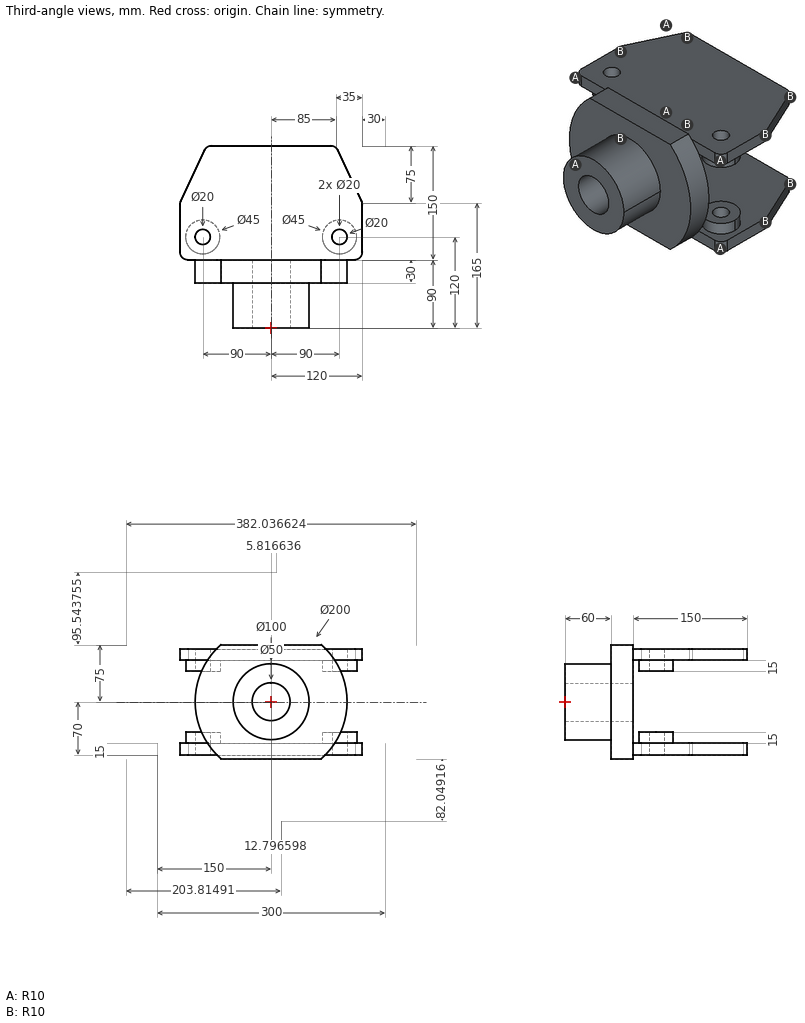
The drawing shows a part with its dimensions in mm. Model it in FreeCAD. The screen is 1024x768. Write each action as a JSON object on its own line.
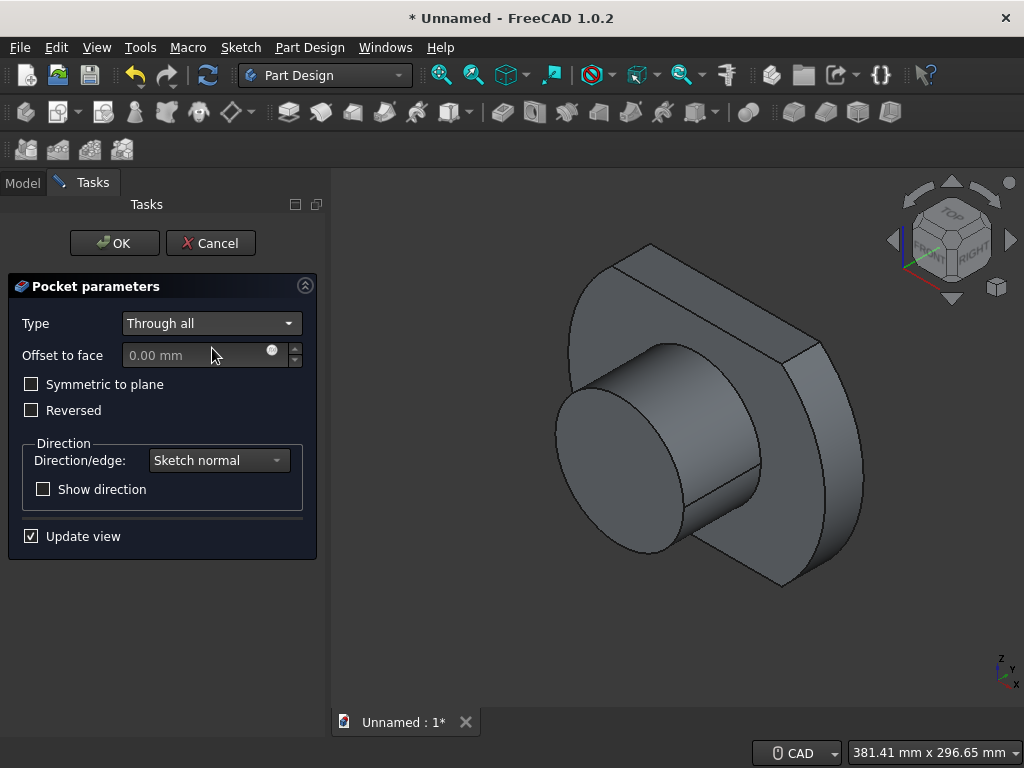
{"action": "left_click", "coordinate": [115, 243]}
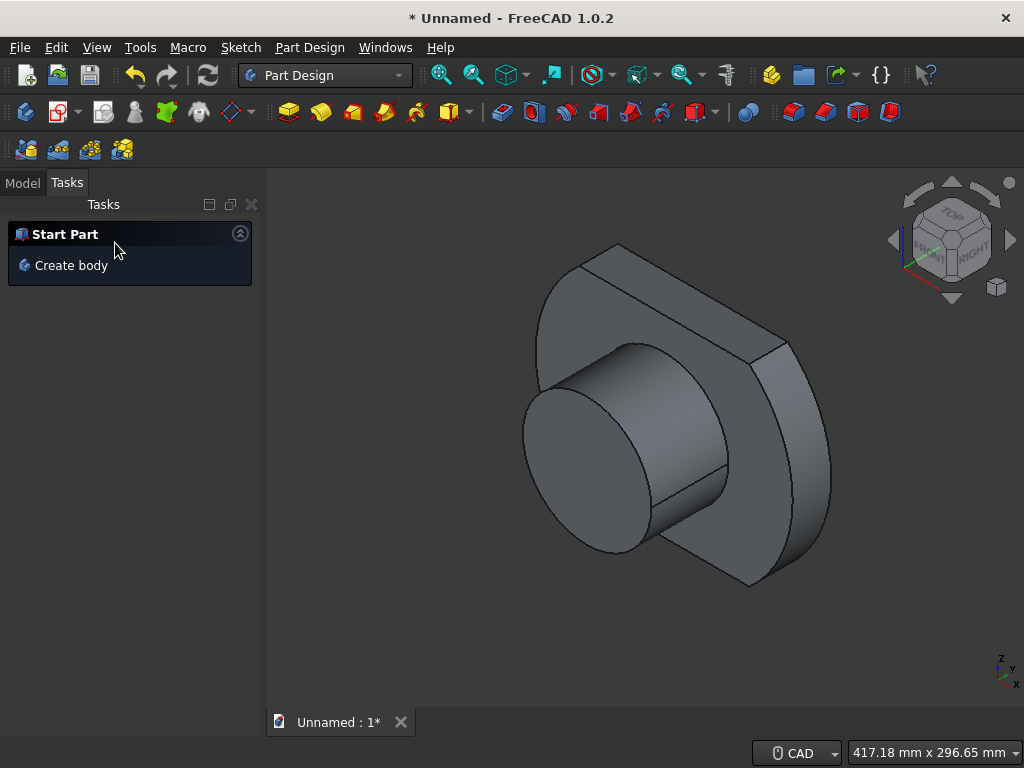
{"action": "key", "text": "4"}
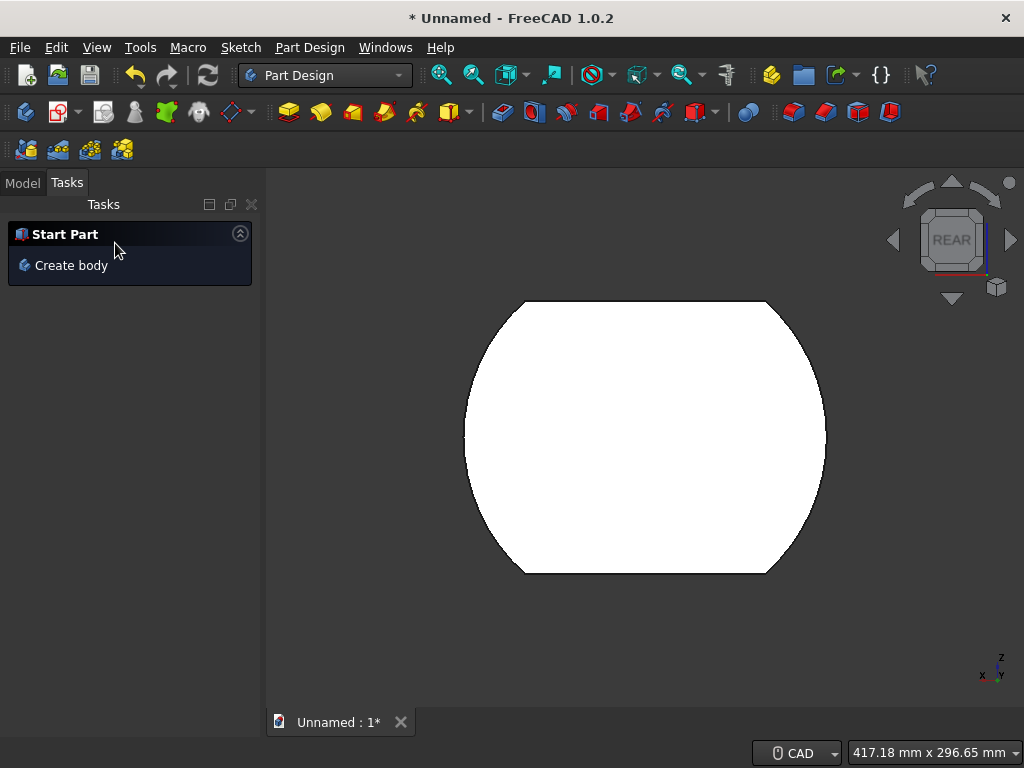
{"action": "left_click", "coordinate": [645, 436]}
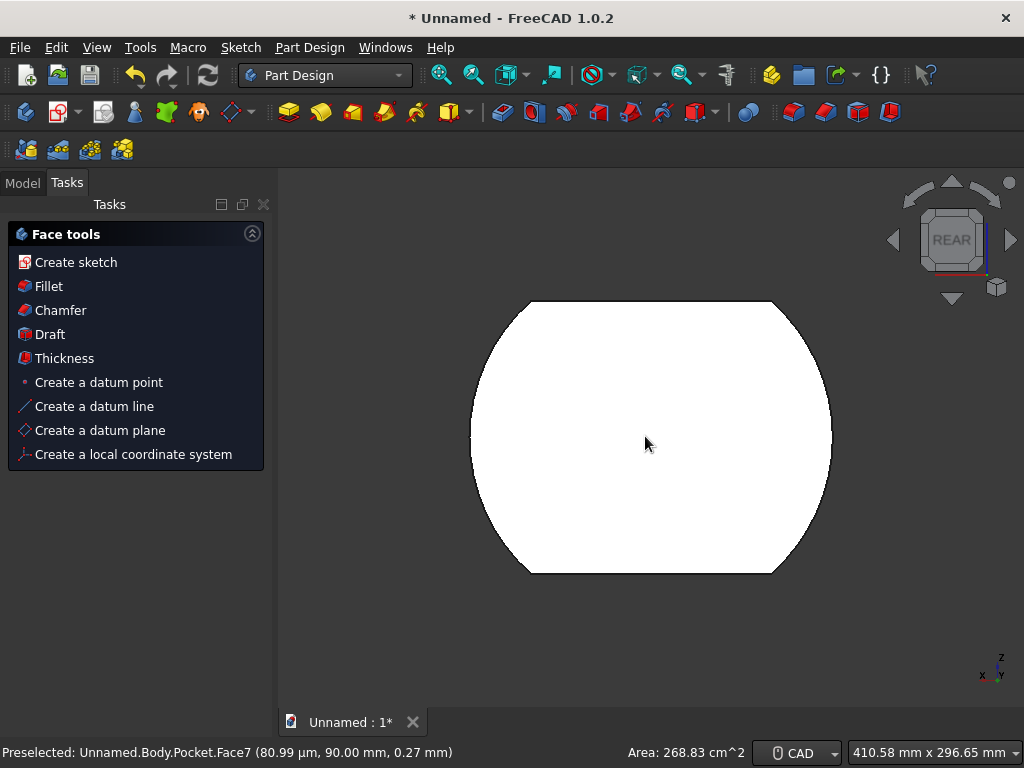
{"action": "left_click", "coordinate": [58, 112]}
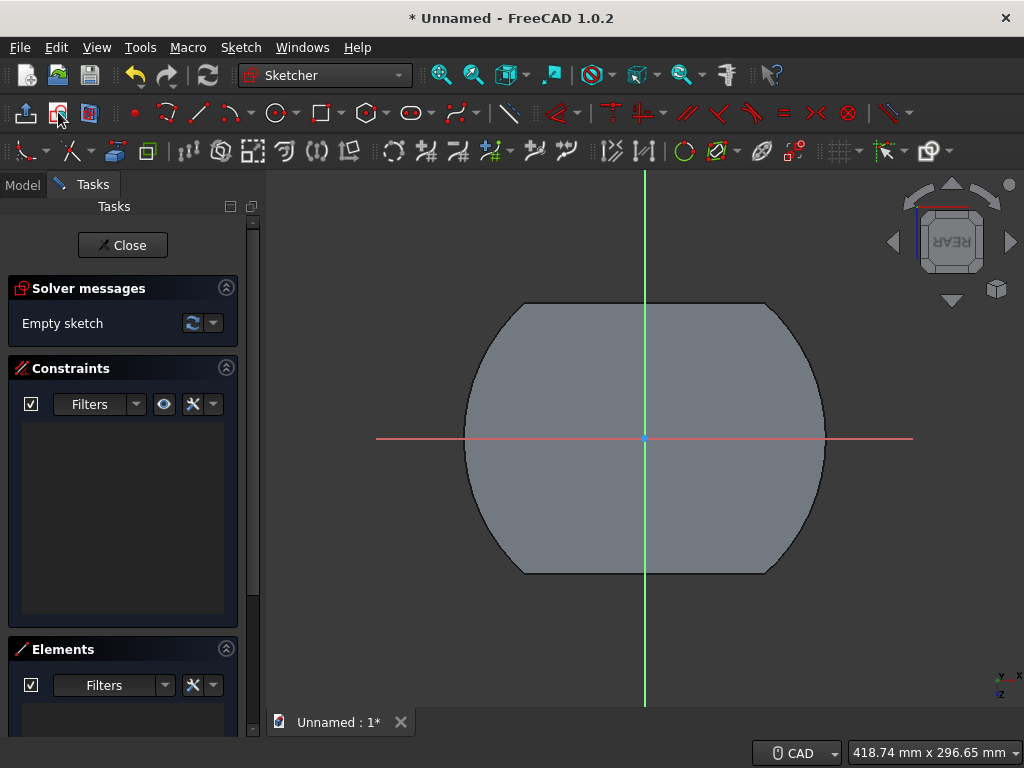
{"action": "scroll", "coordinate": [438, 438], "scroll_direction": "down", "scroll_amount": 2}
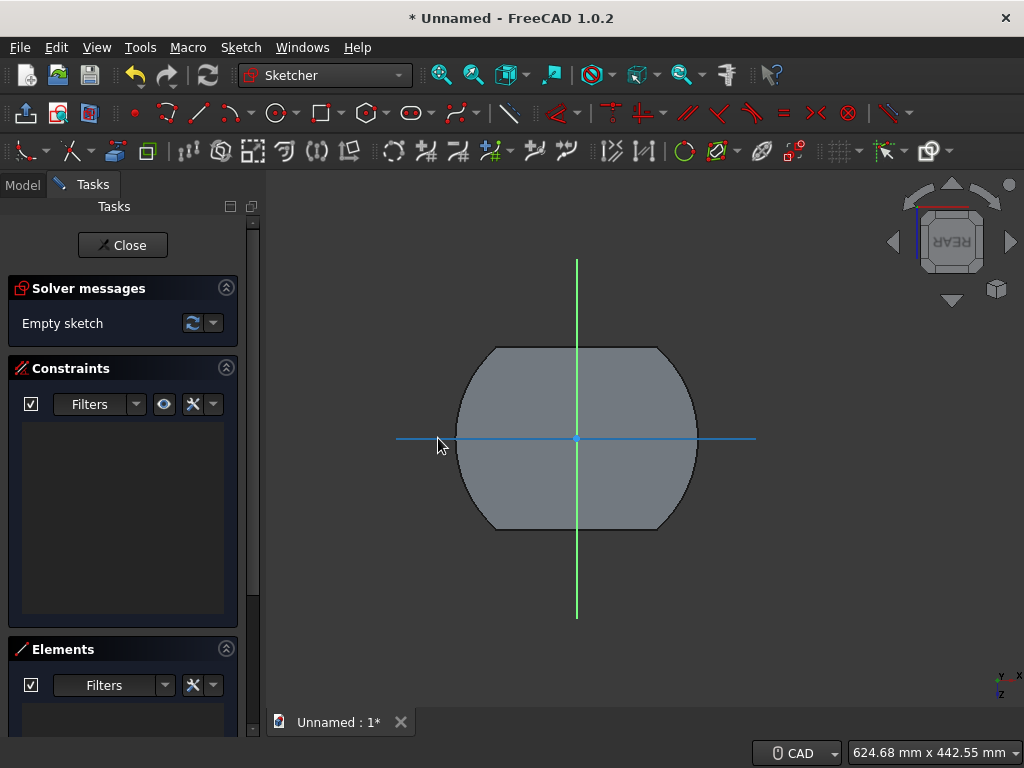
{"action": "left_click", "coordinate": [322, 114]}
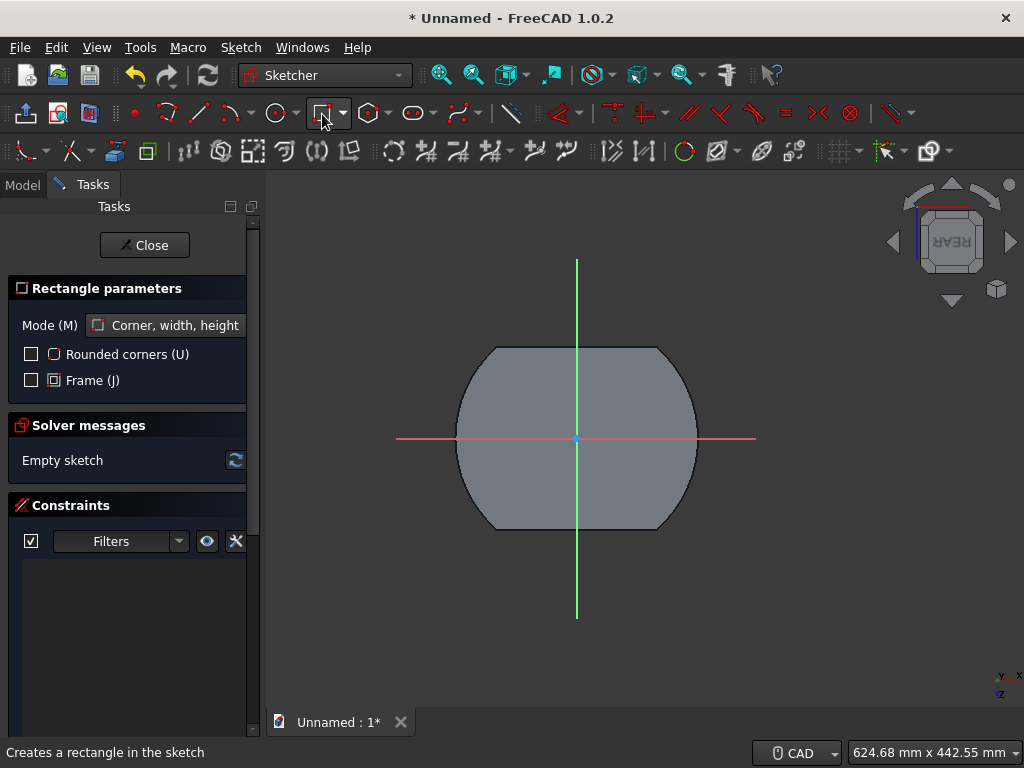
{"action": "left_click", "coordinate": [395, 354]}
{"action": "left_click", "coordinate": [759, 372]}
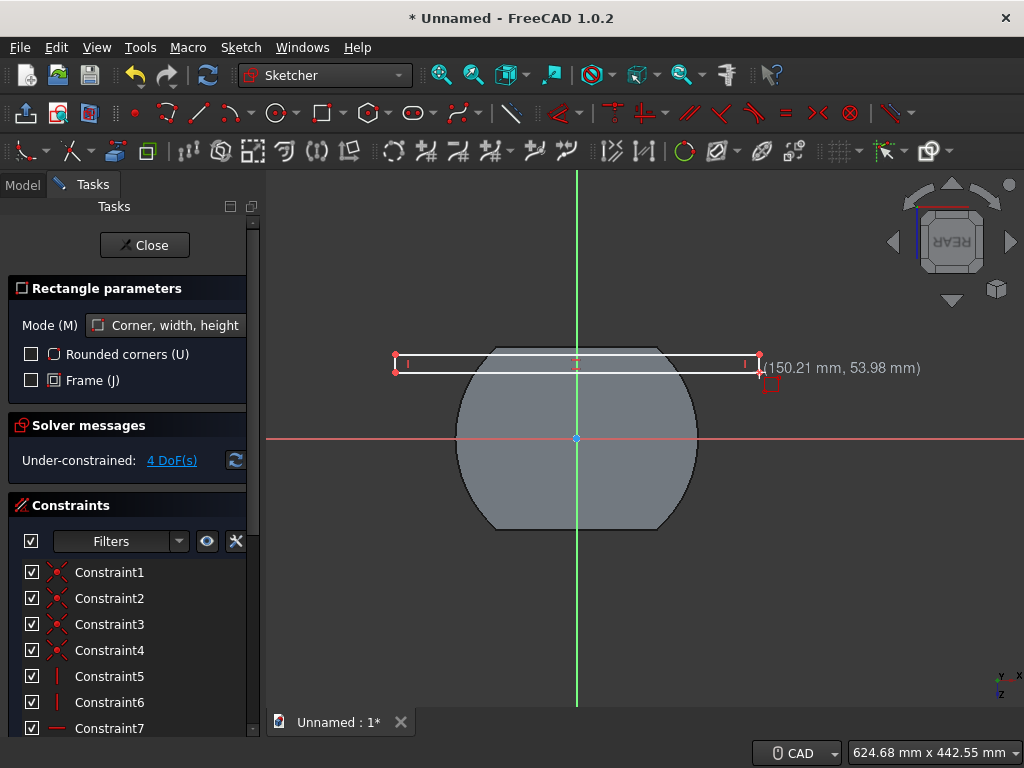
{"action": "left_click", "coordinate": [395, 505]}
{"action": "left_click", "coordinate": [759, 523]}
{"action": "key", "text": "Escape"}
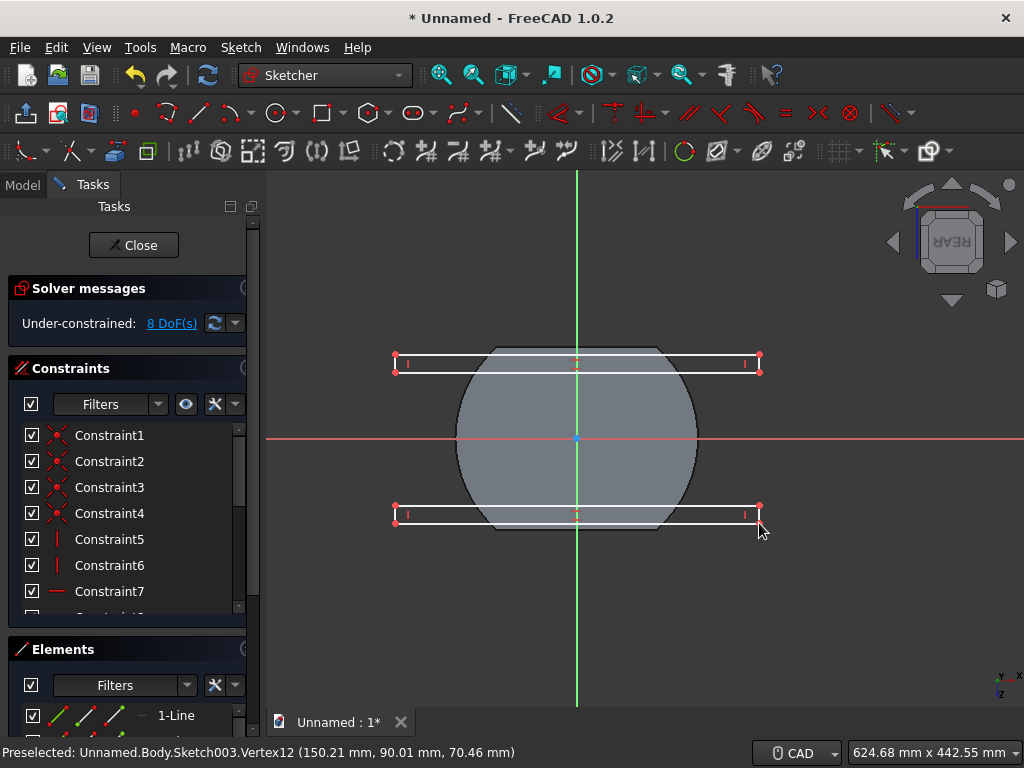
{"action": "left_click", "coordinate": [395, 373]}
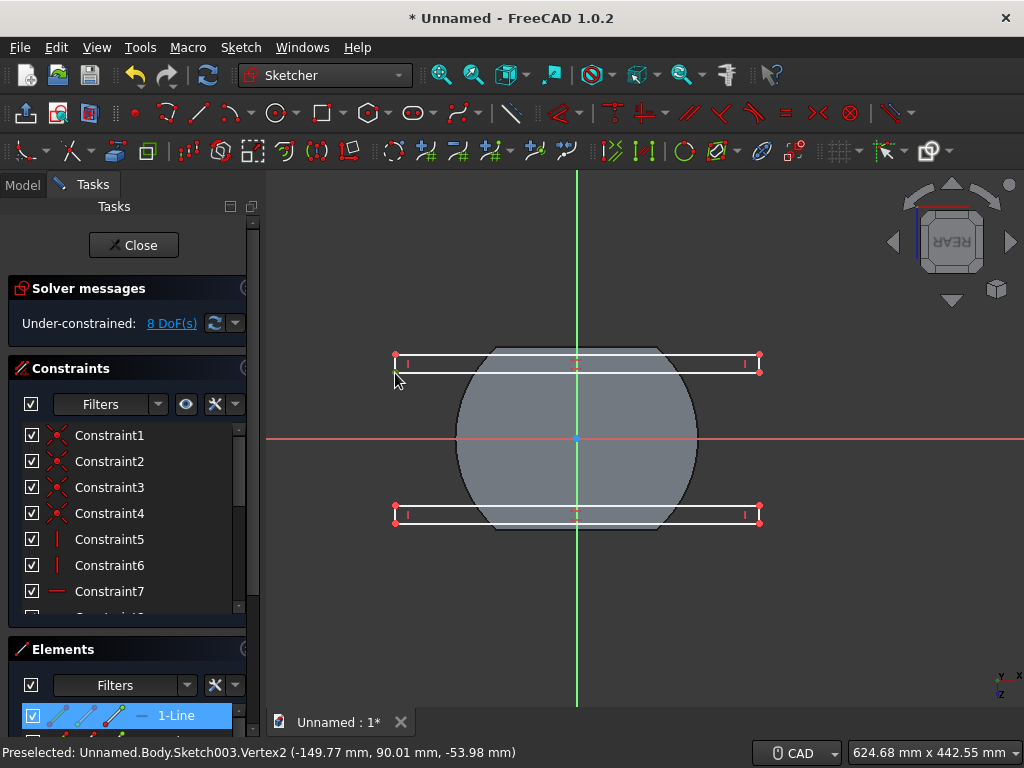
{"action": "left_click", "coordinate": [395, 506]}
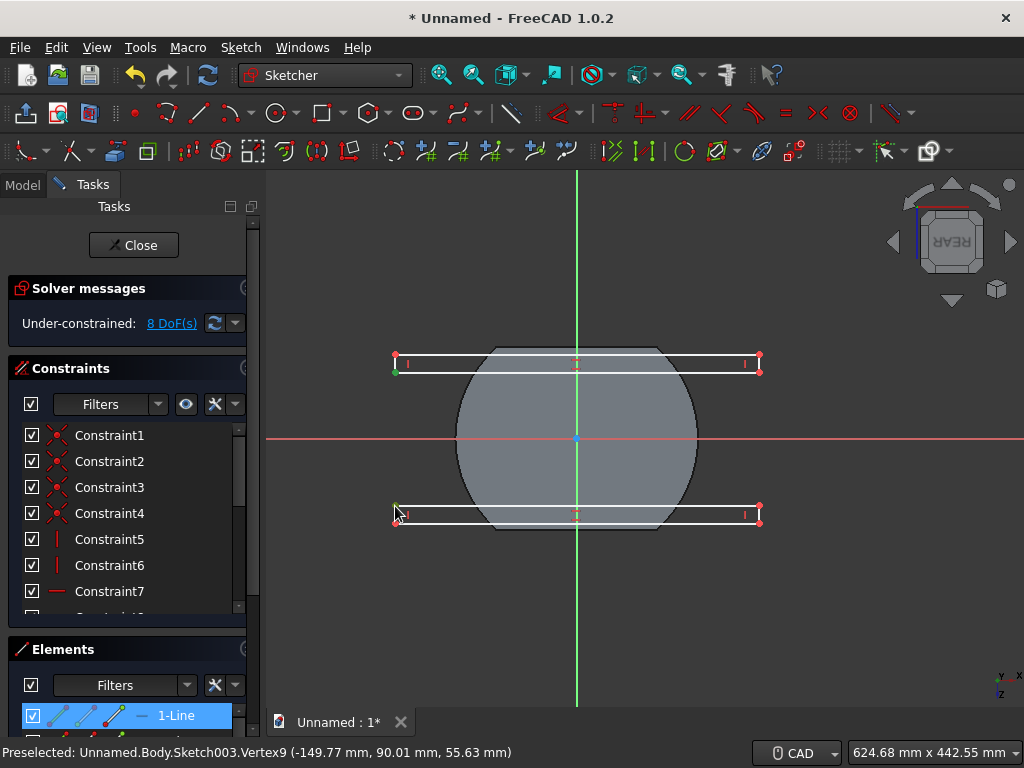
{"action": "left_click", "coordinate": [334, 439]}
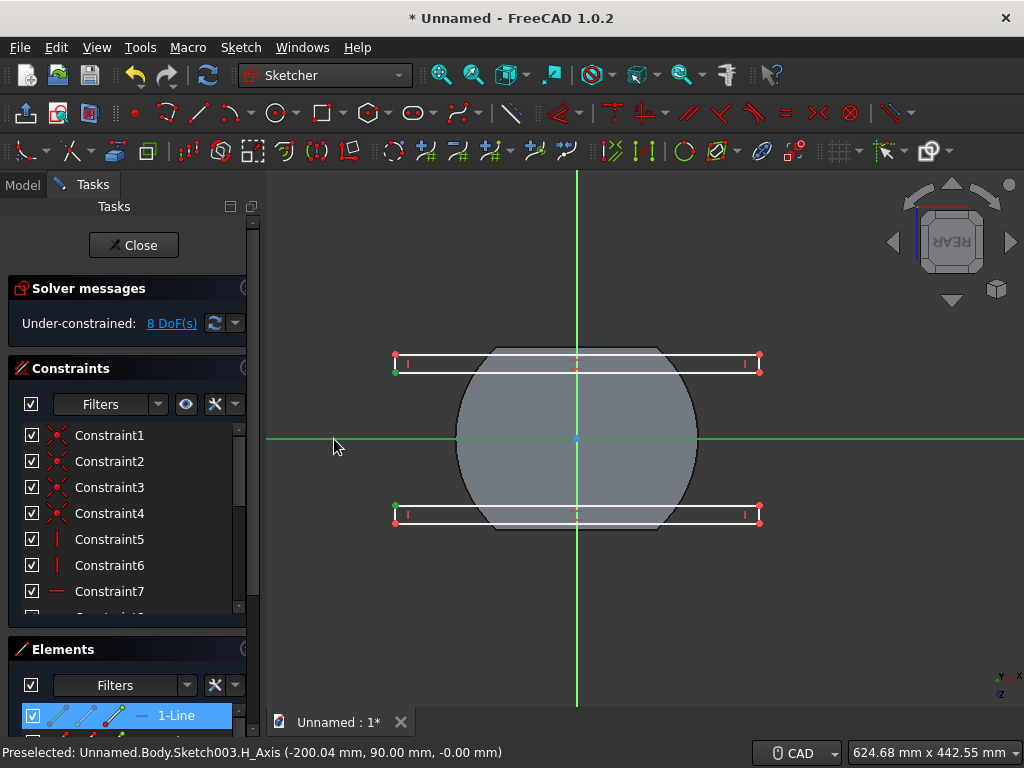
{"action": "left_click", "coordinate": [818, 114]}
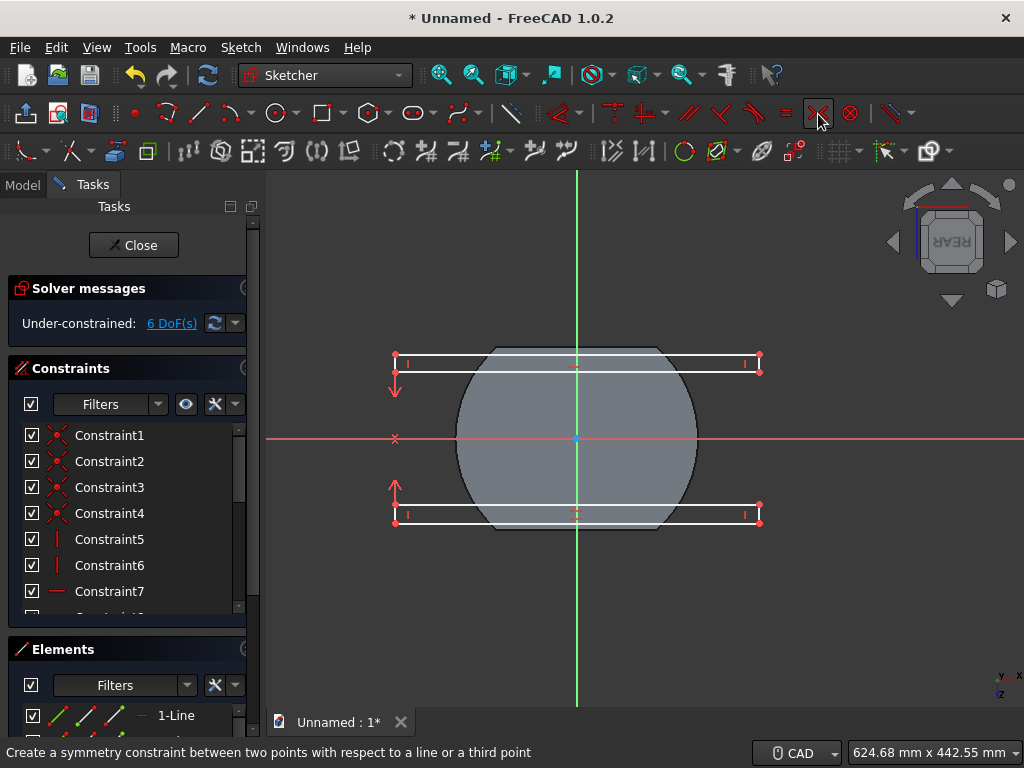
{"action": "left_click", "coordinate": [759, 355]}